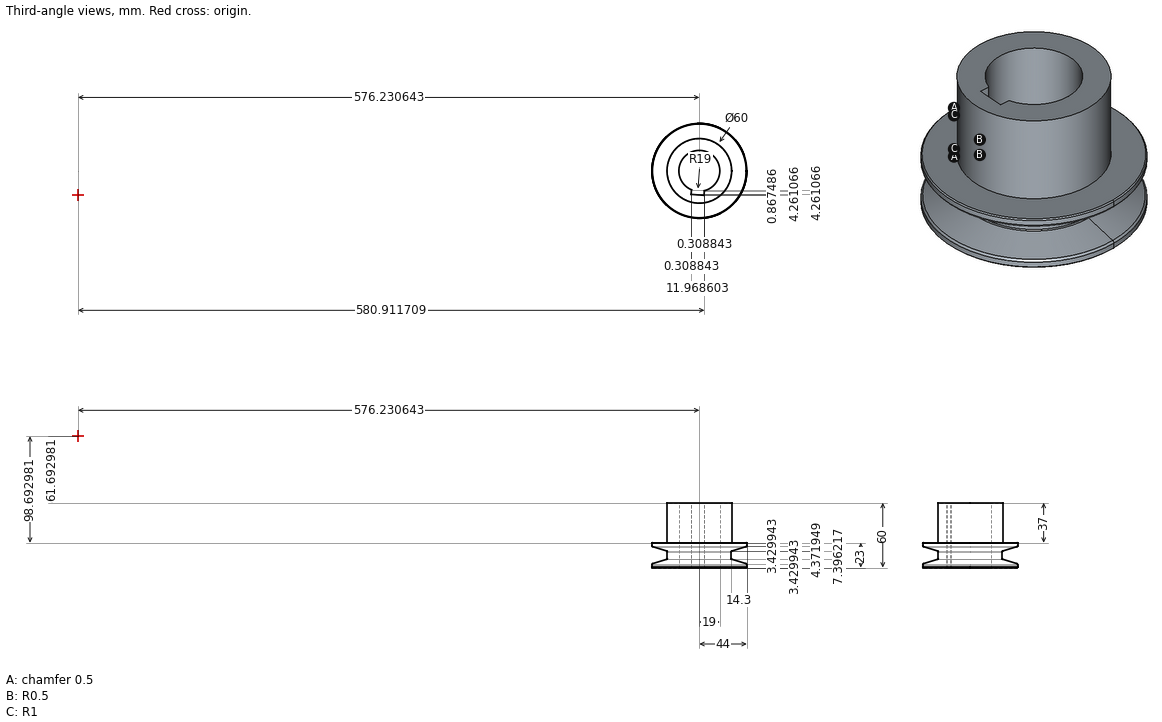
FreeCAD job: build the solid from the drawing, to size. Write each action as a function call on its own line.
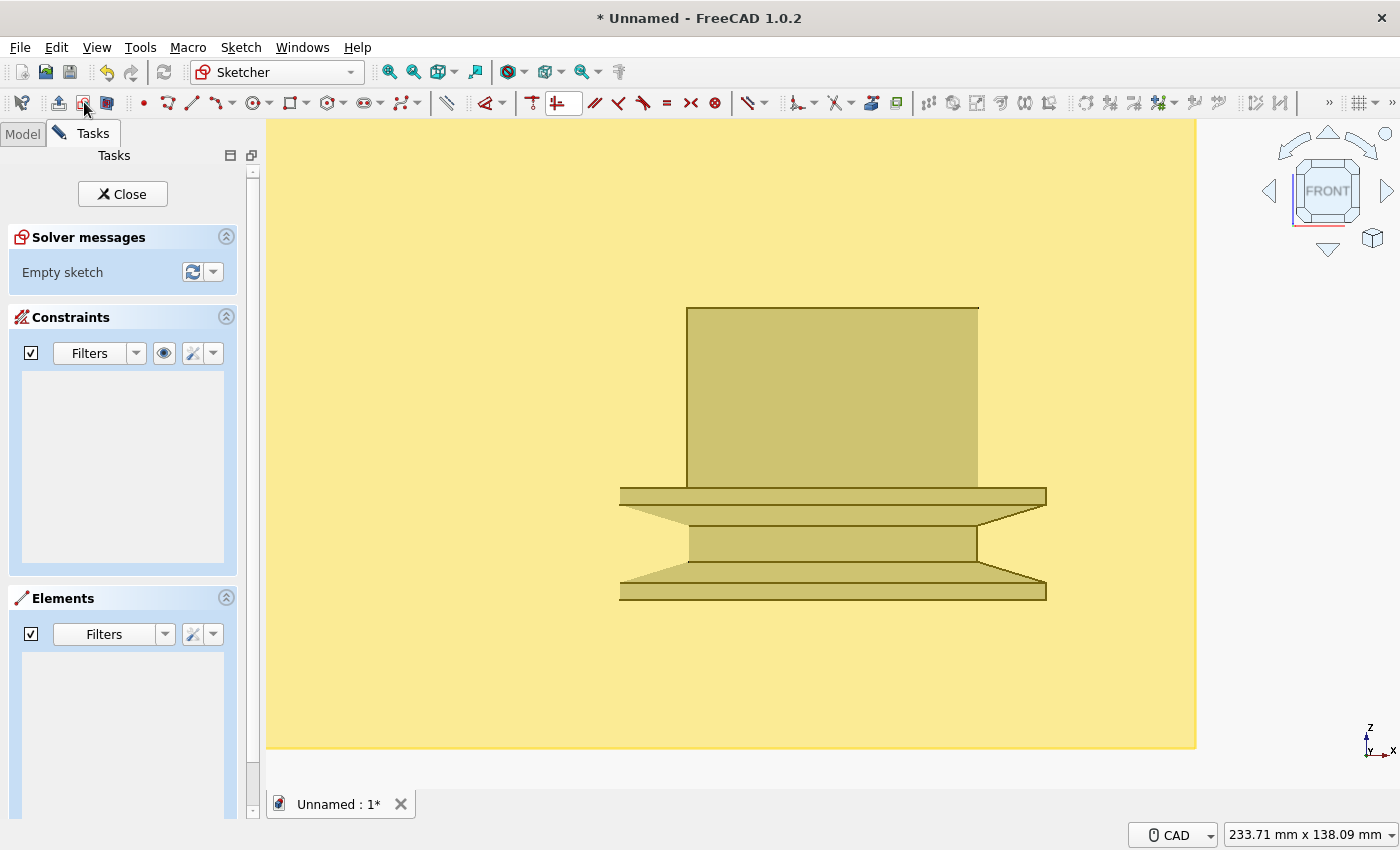
key(g)
key(r)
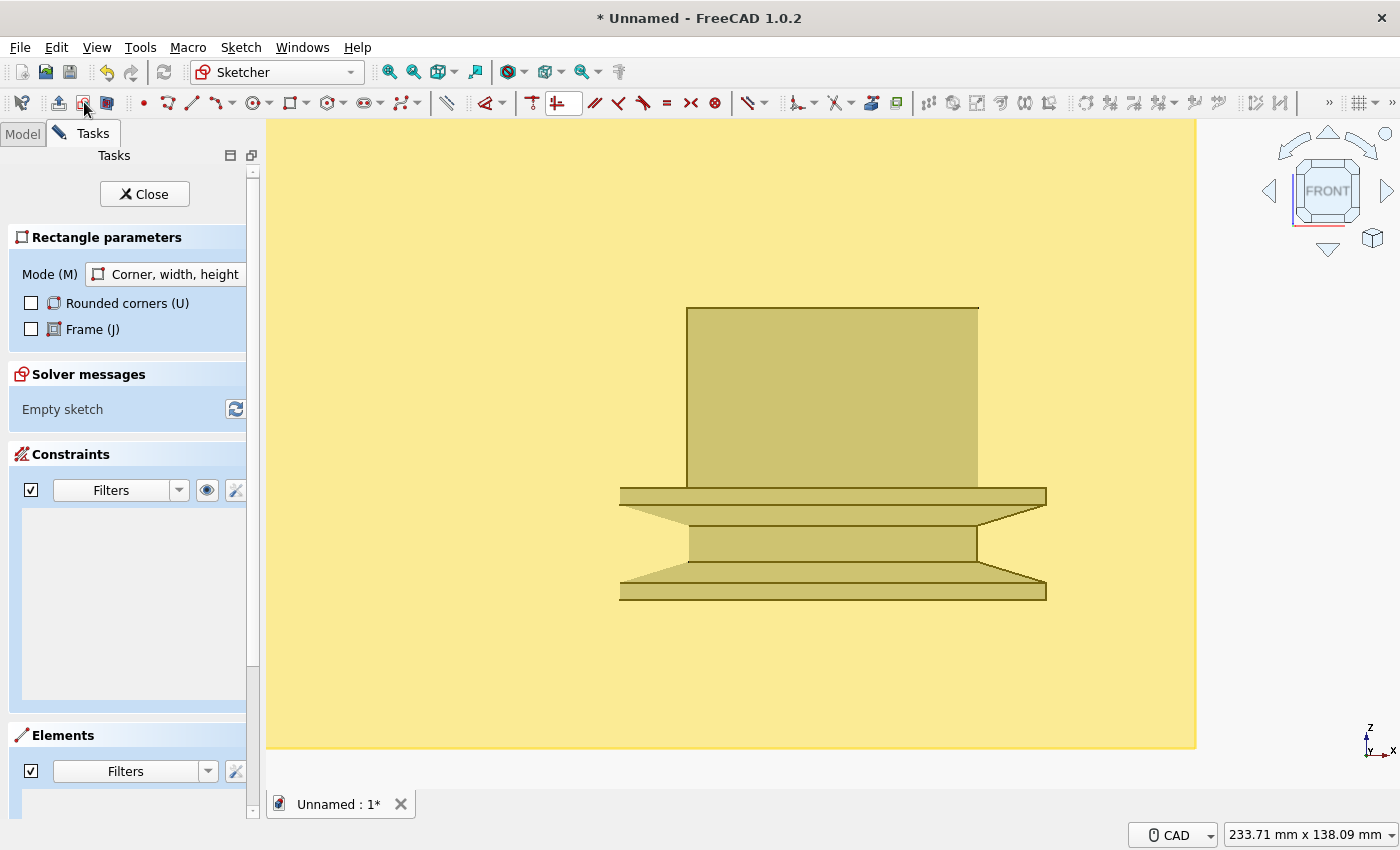
click(833, 308)
click(925, 600)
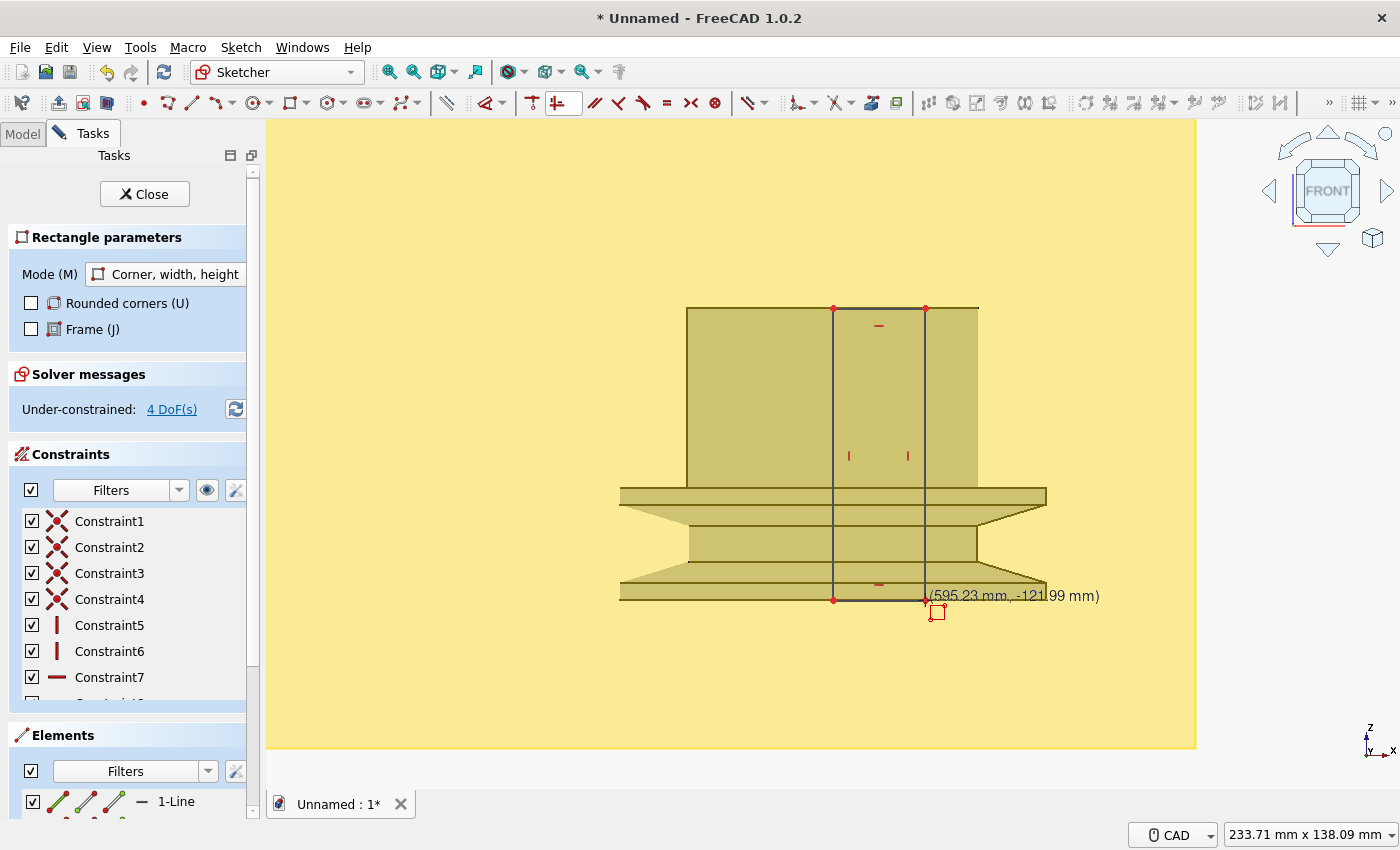
click(192, 104)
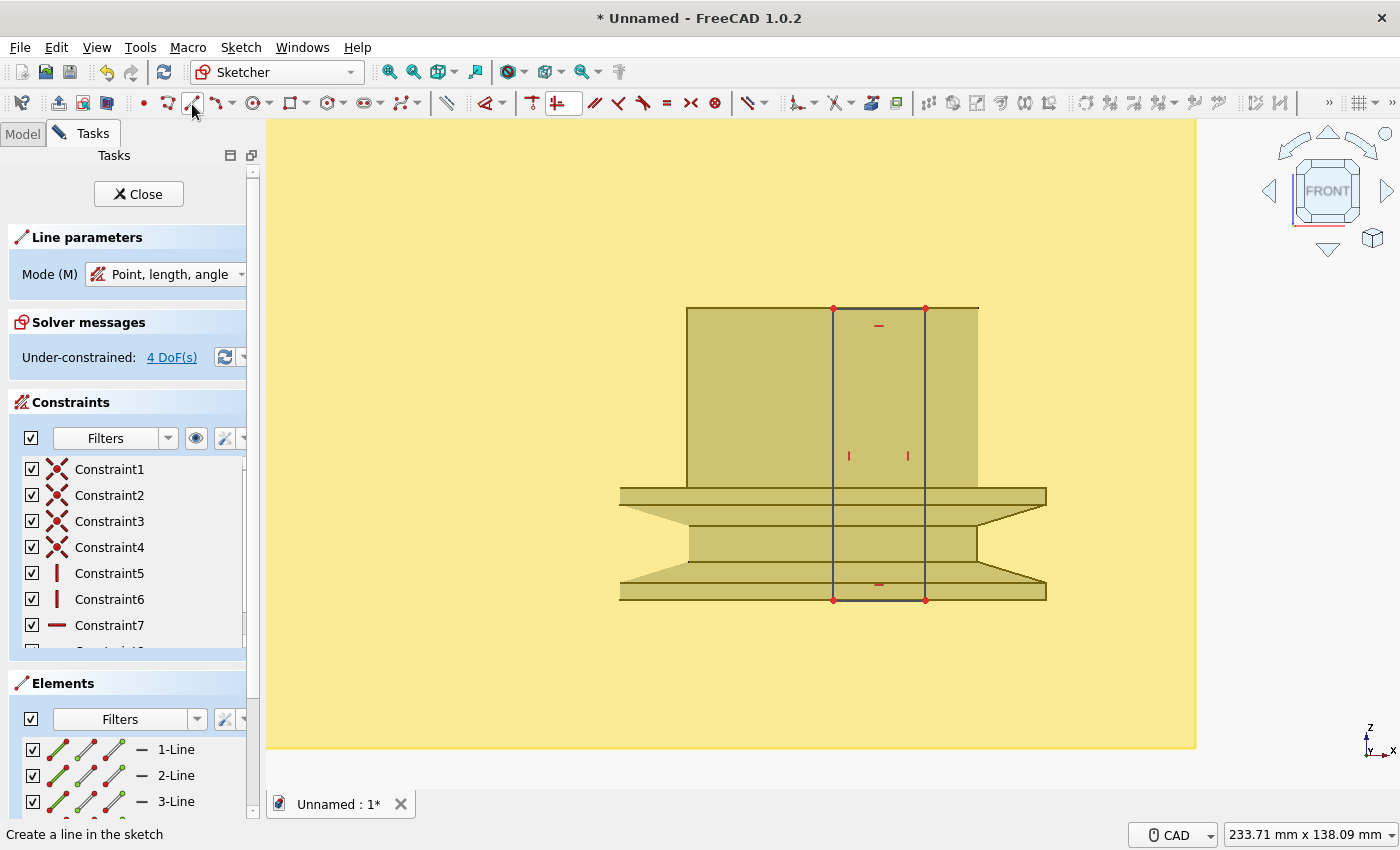
click(833, 629)
click(833, 716)
key(Escape)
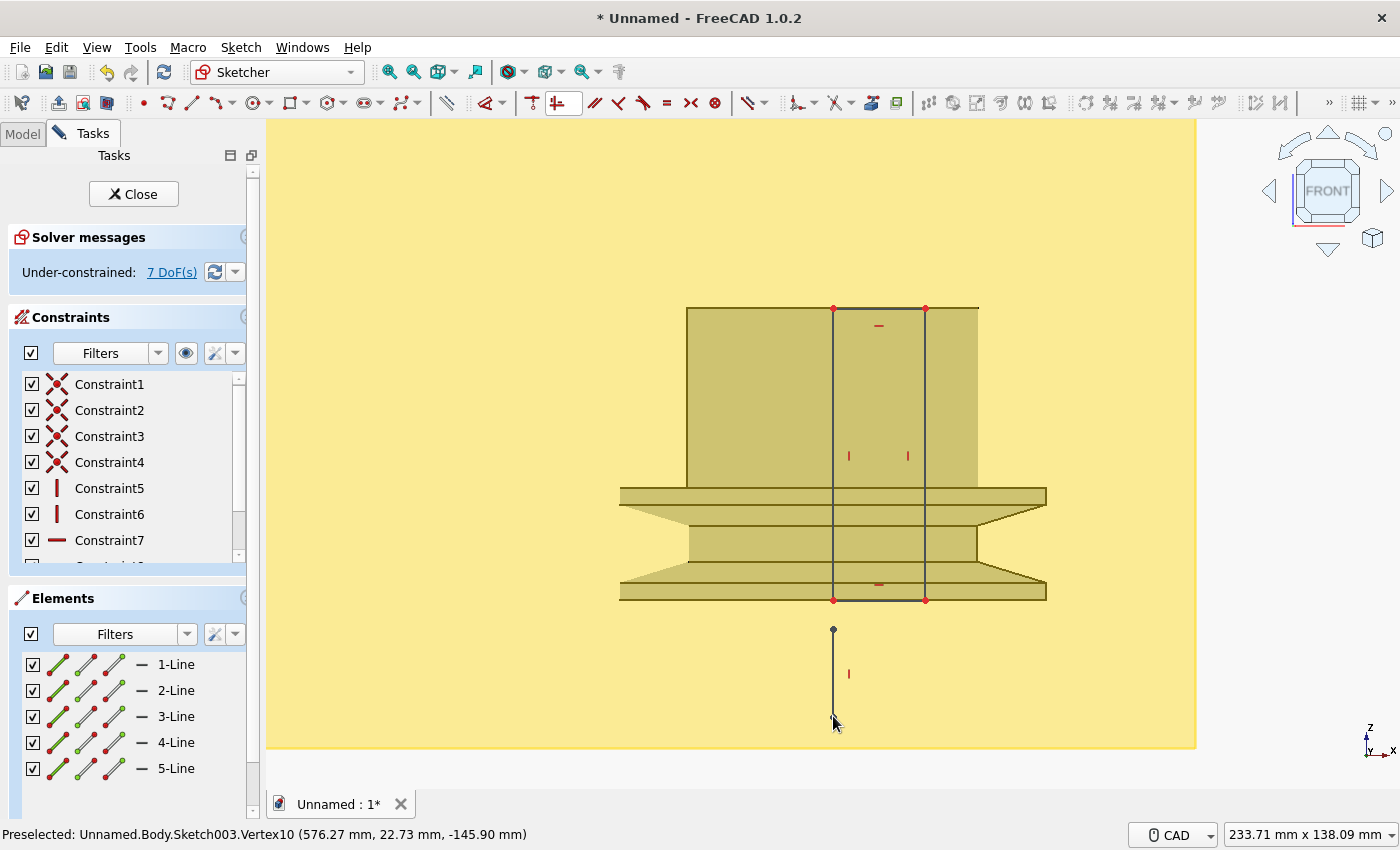
click(833, 656)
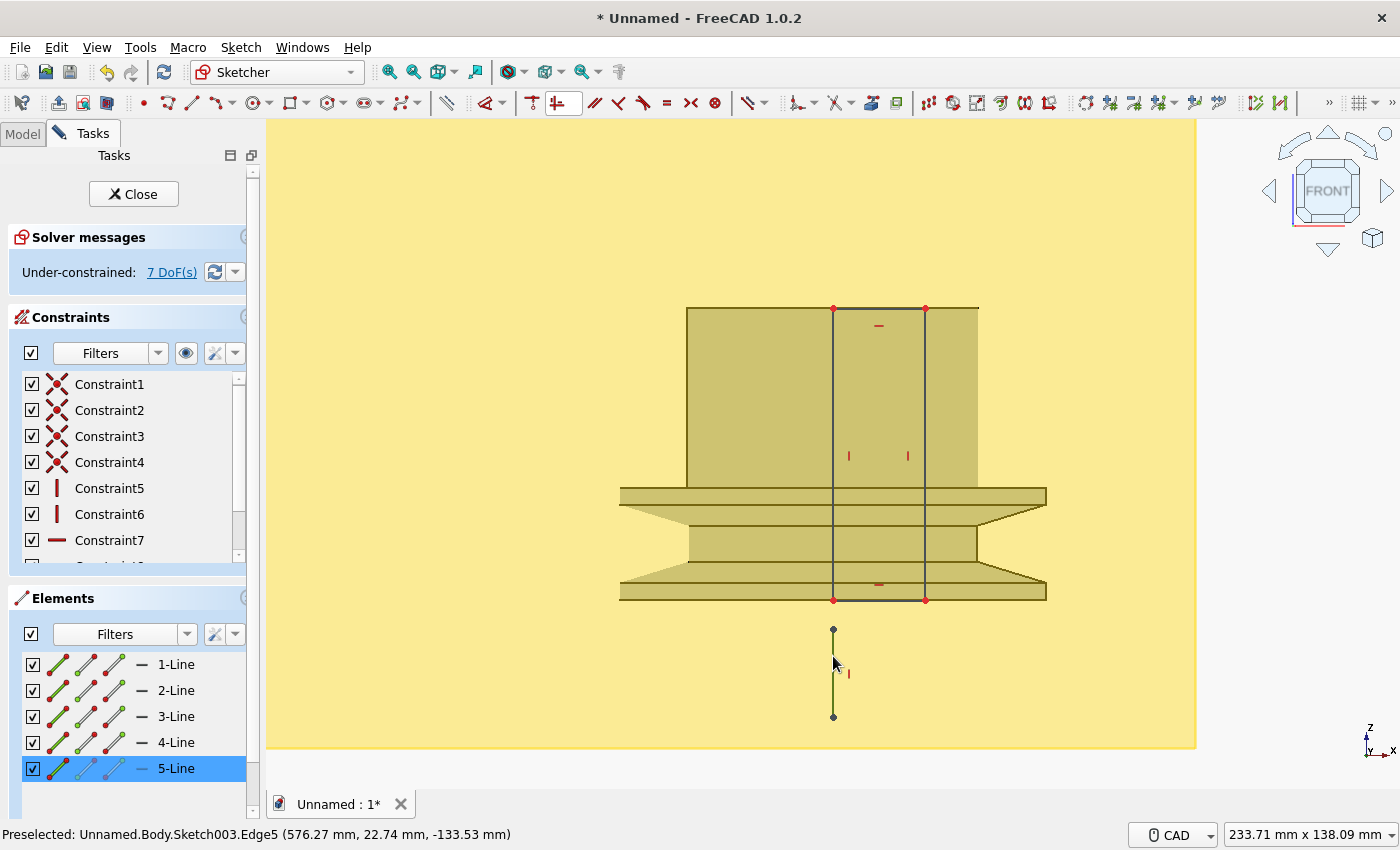
key(g)
key(n)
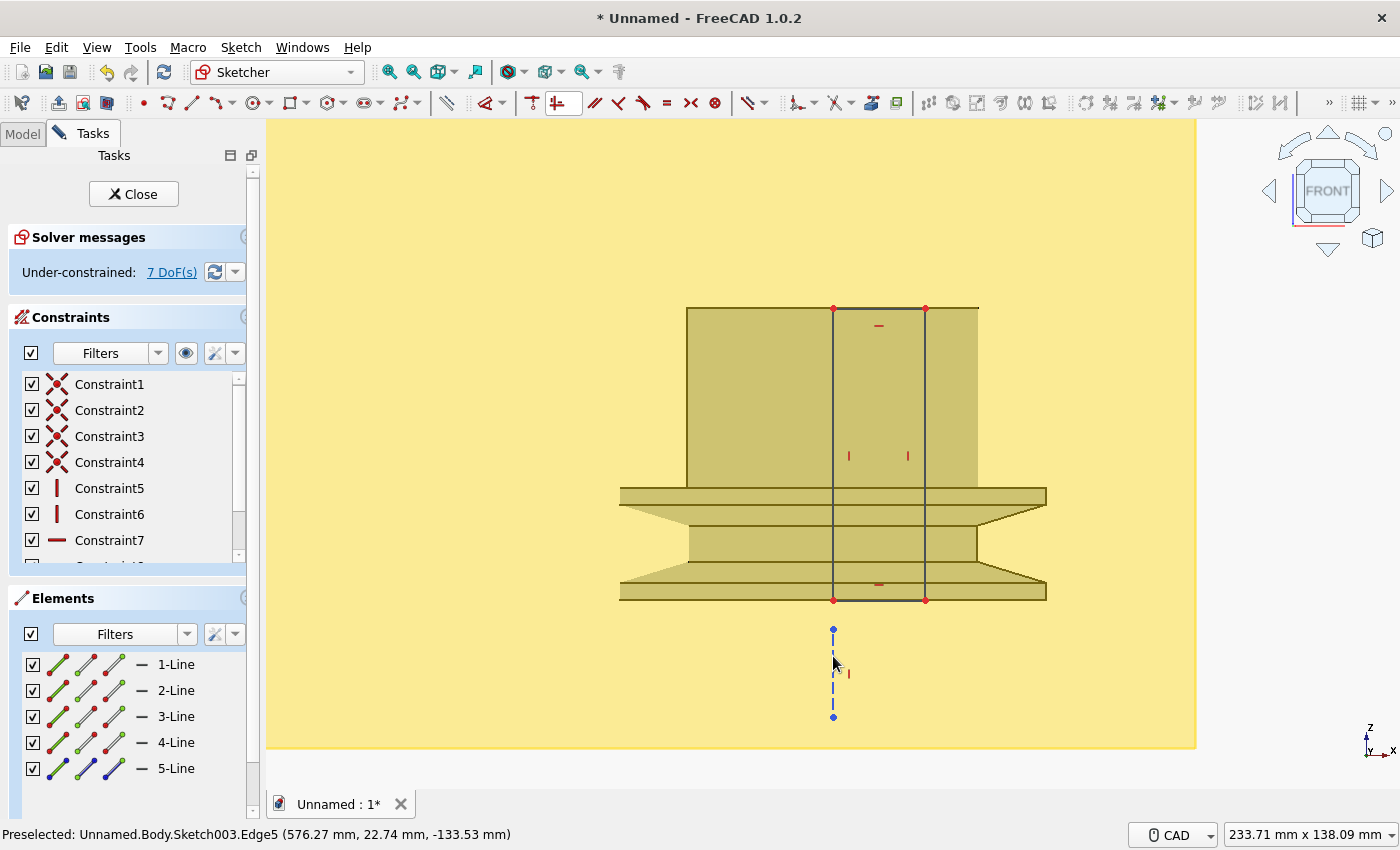
click(486, 104)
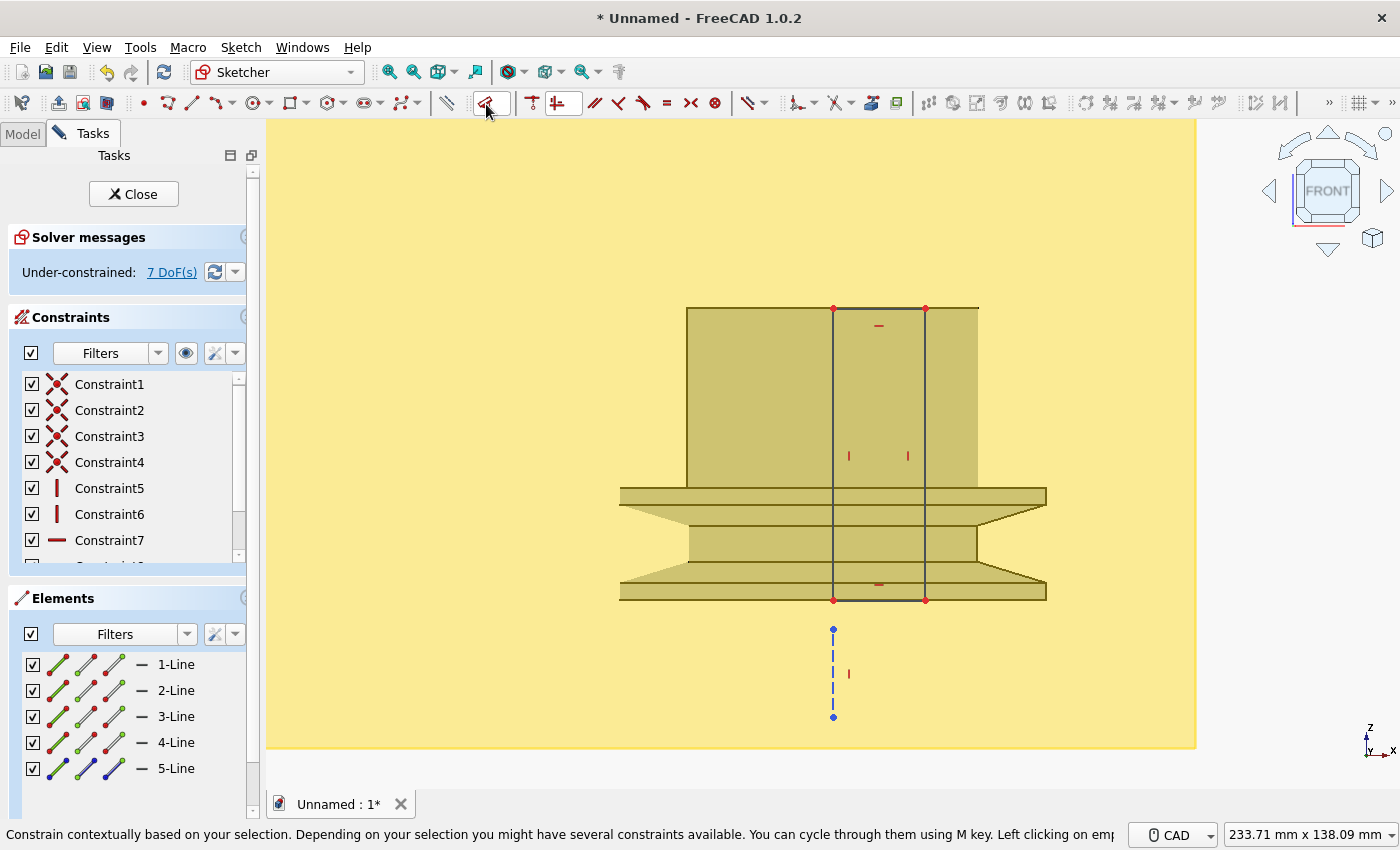
click(833, 397)
click(799, 455)